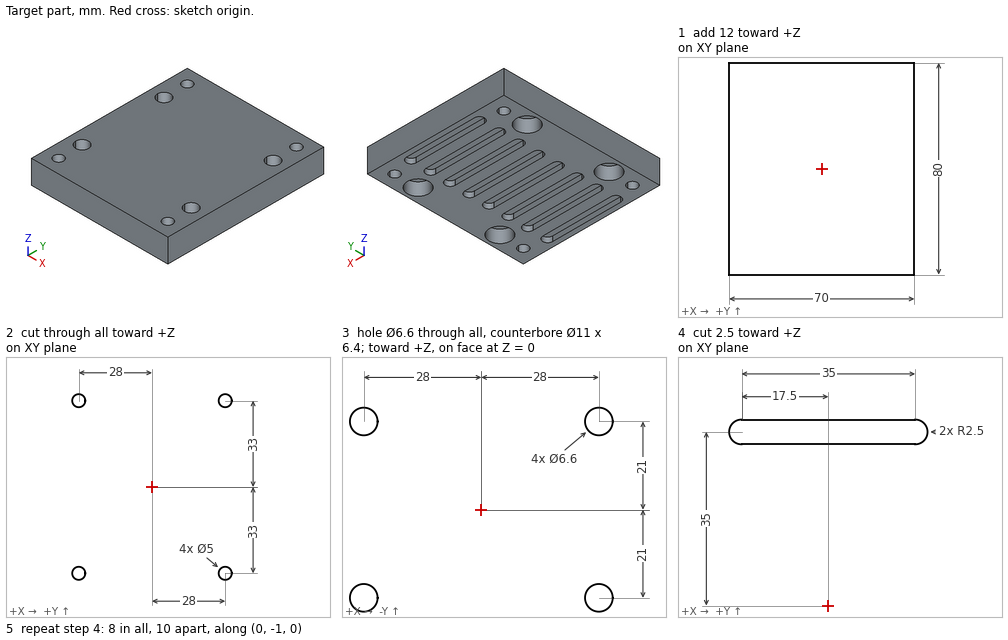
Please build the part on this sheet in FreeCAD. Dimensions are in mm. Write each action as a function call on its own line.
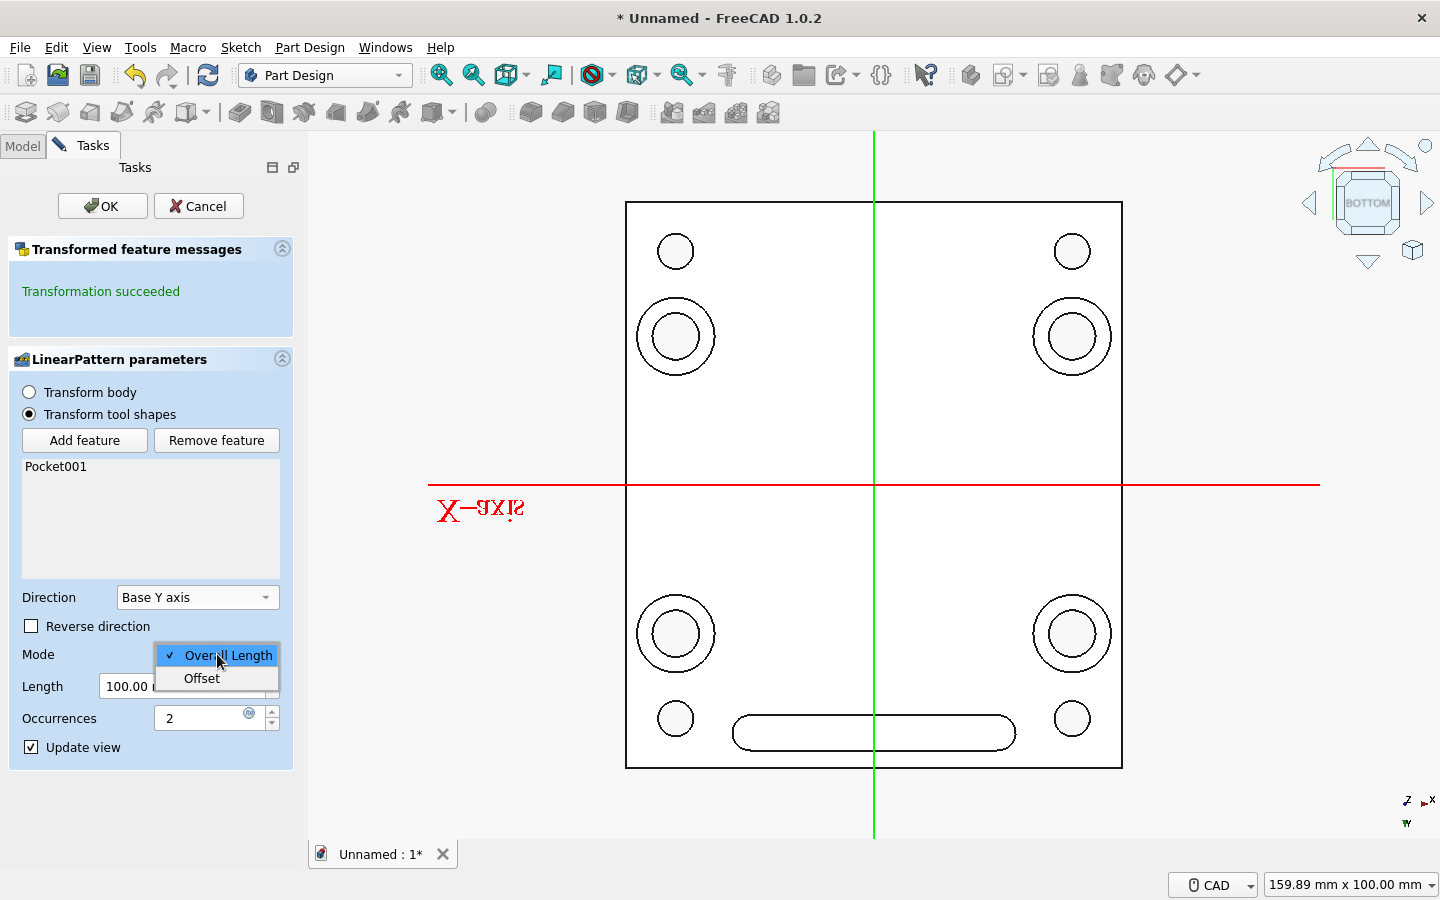
click(216, 678)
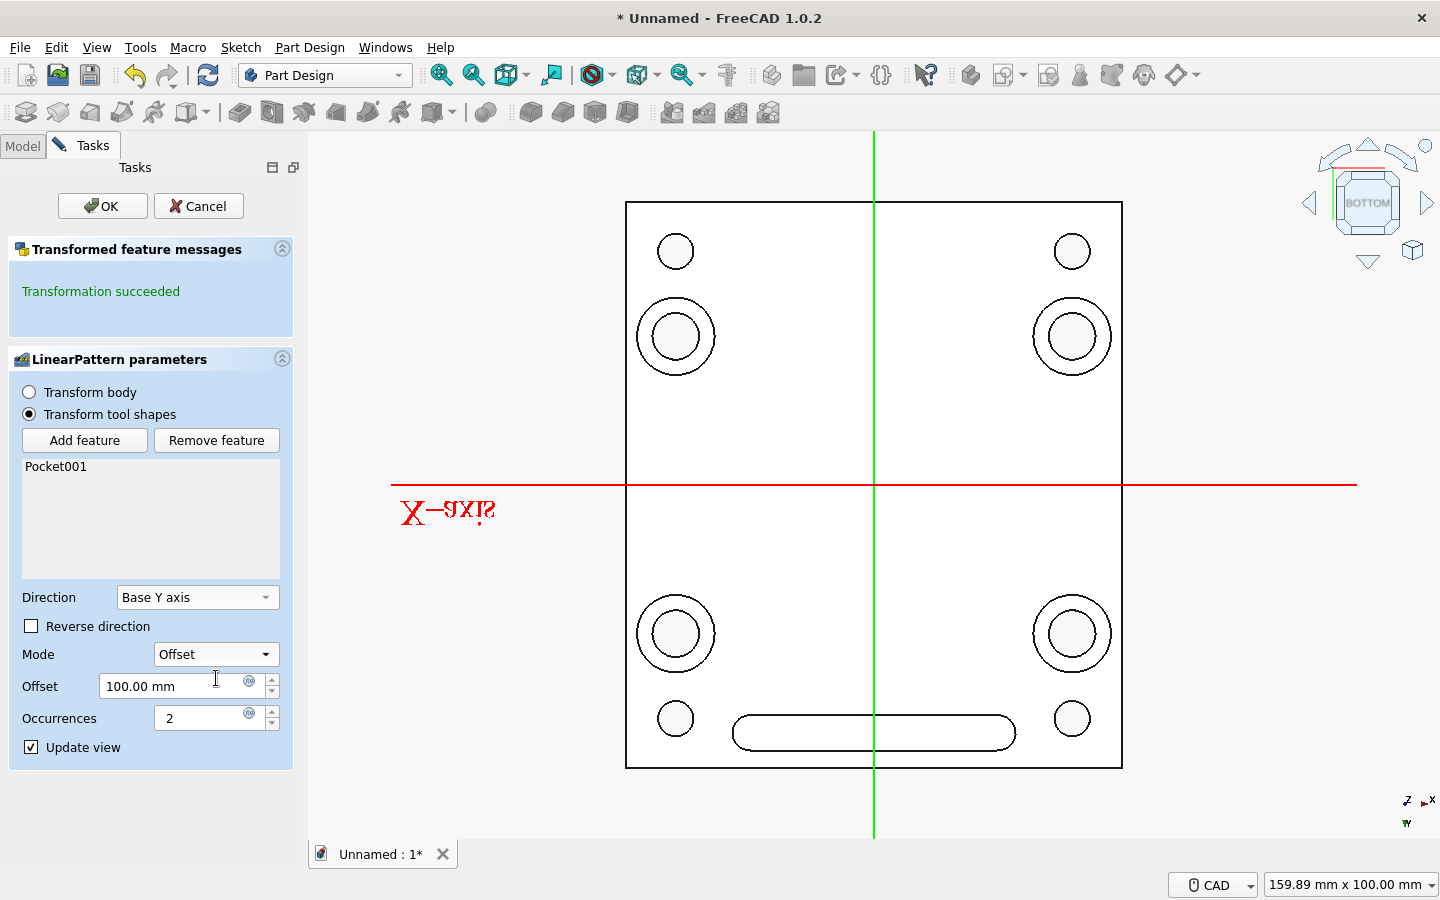
triple_click(182, 686)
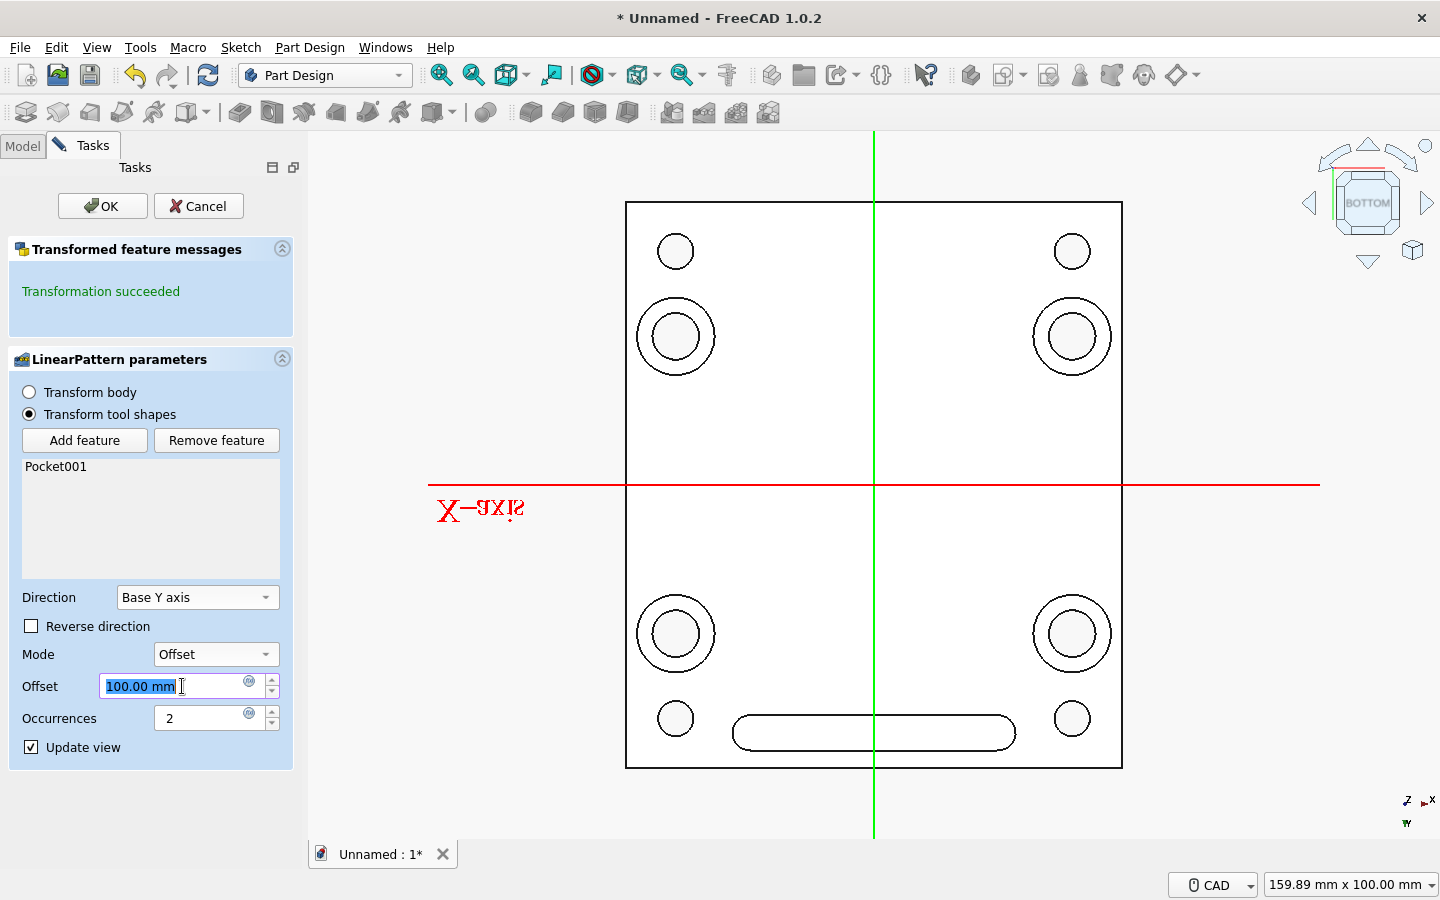
text(10)
key(Tab)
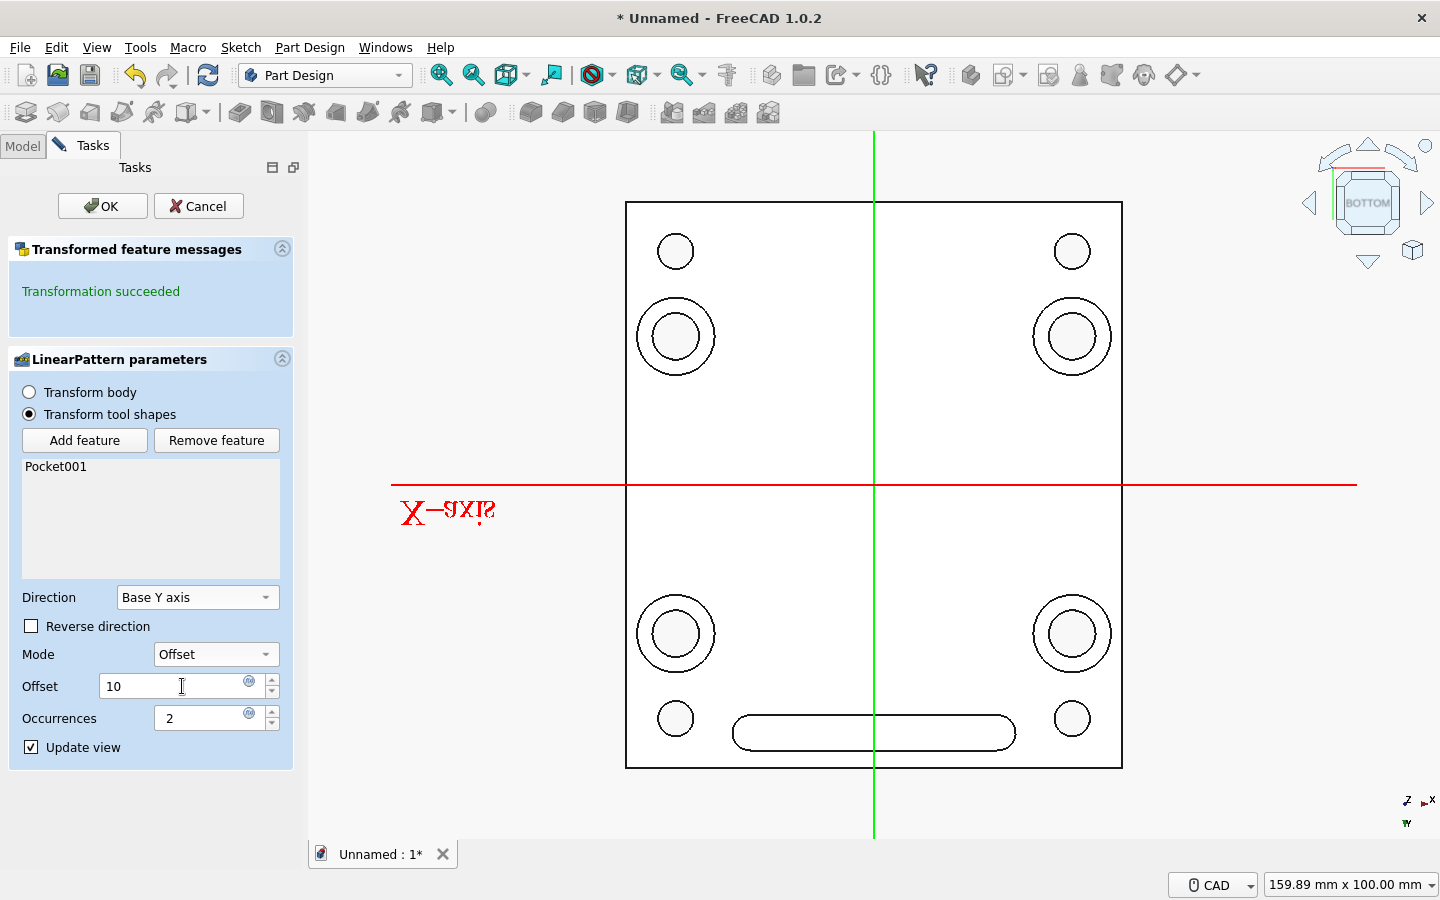
triple_click(209, 718)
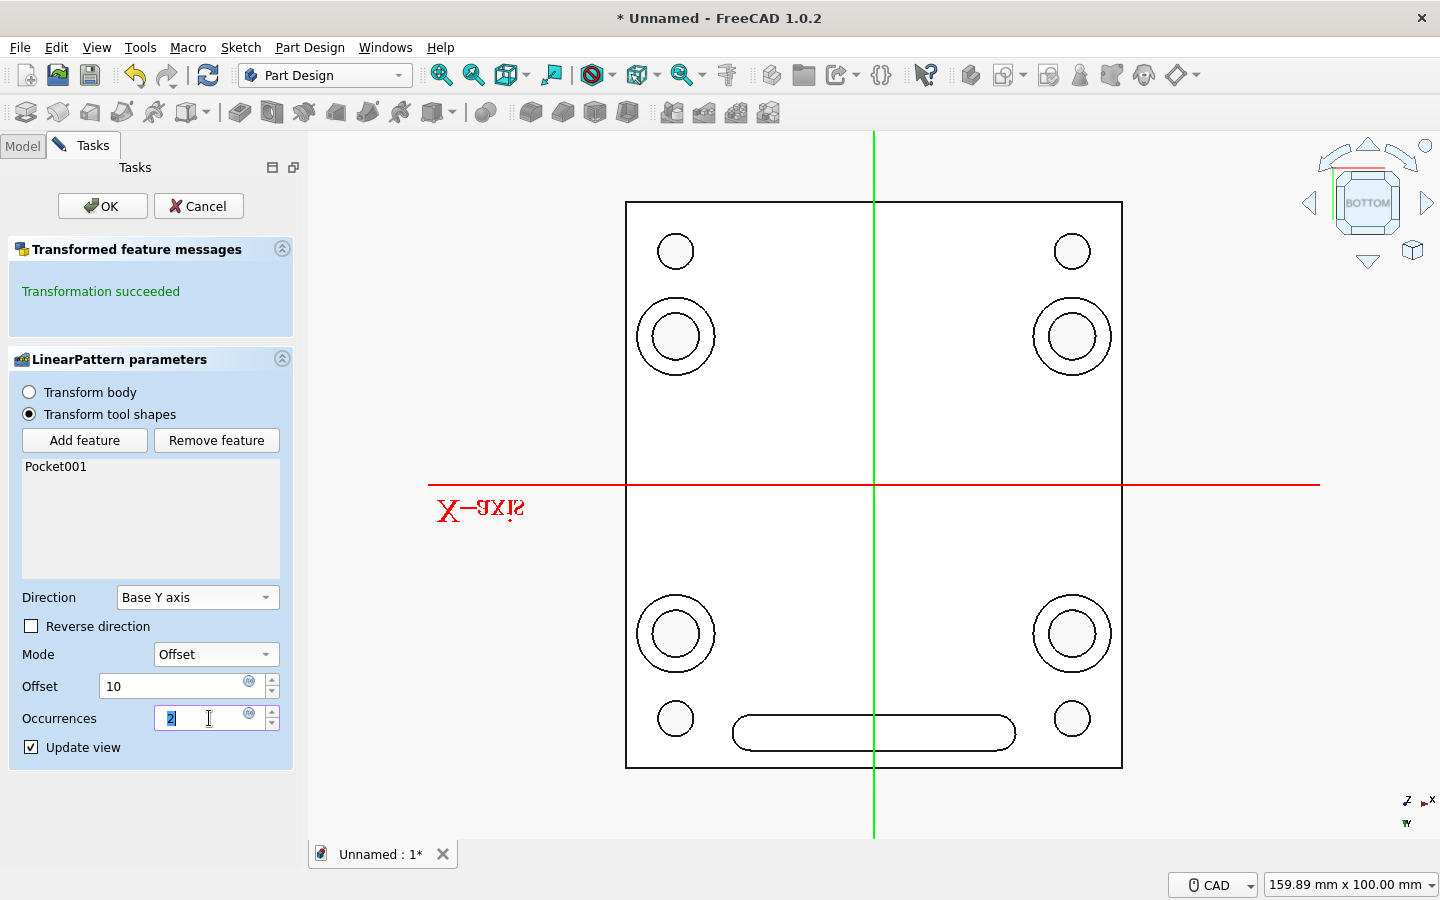
text(8)
key(Tab)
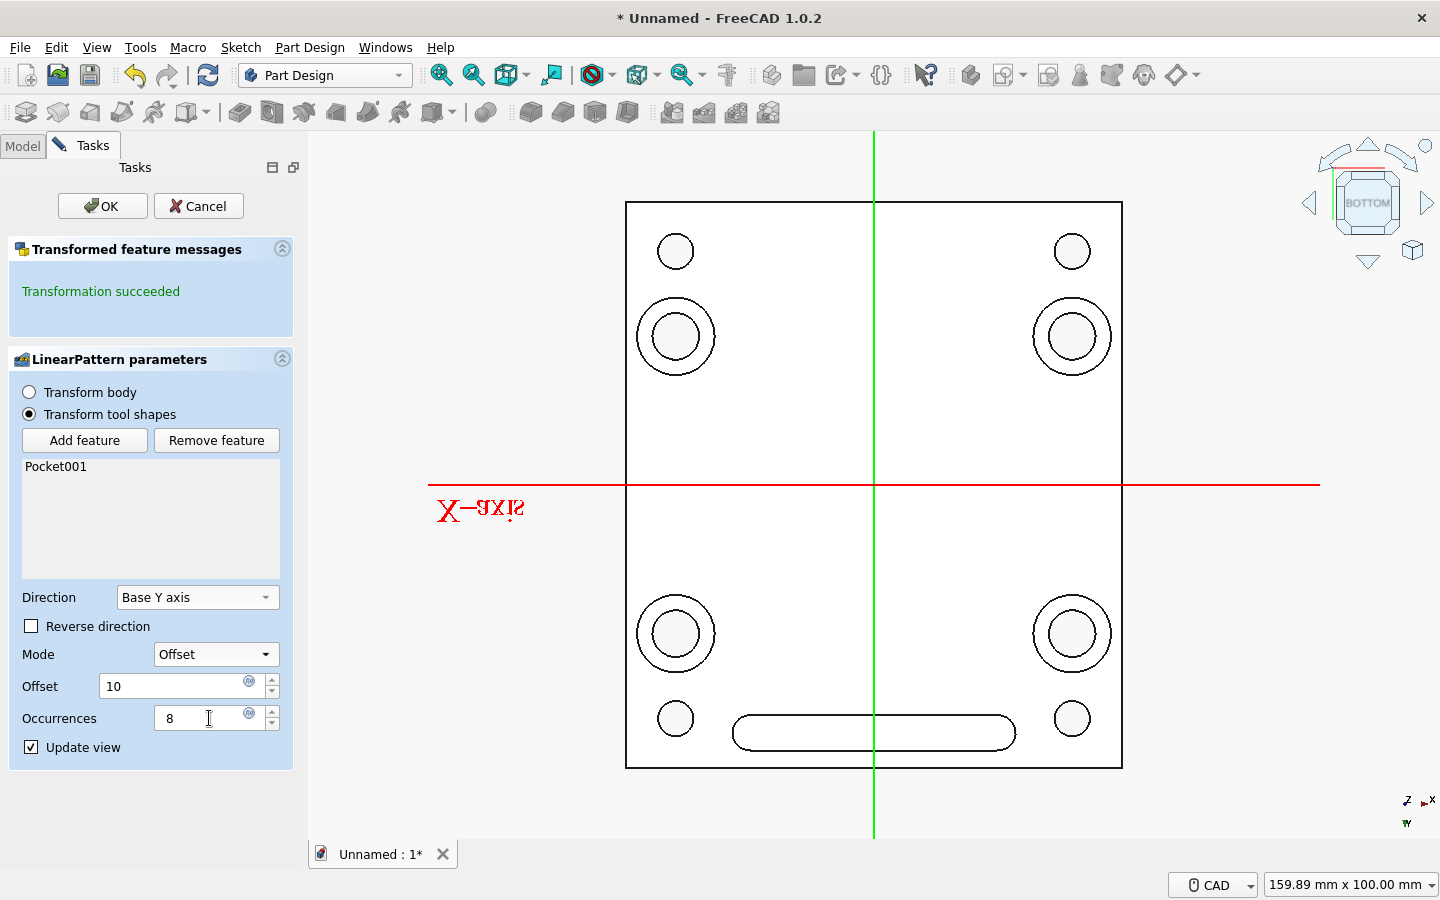
click(30, 626)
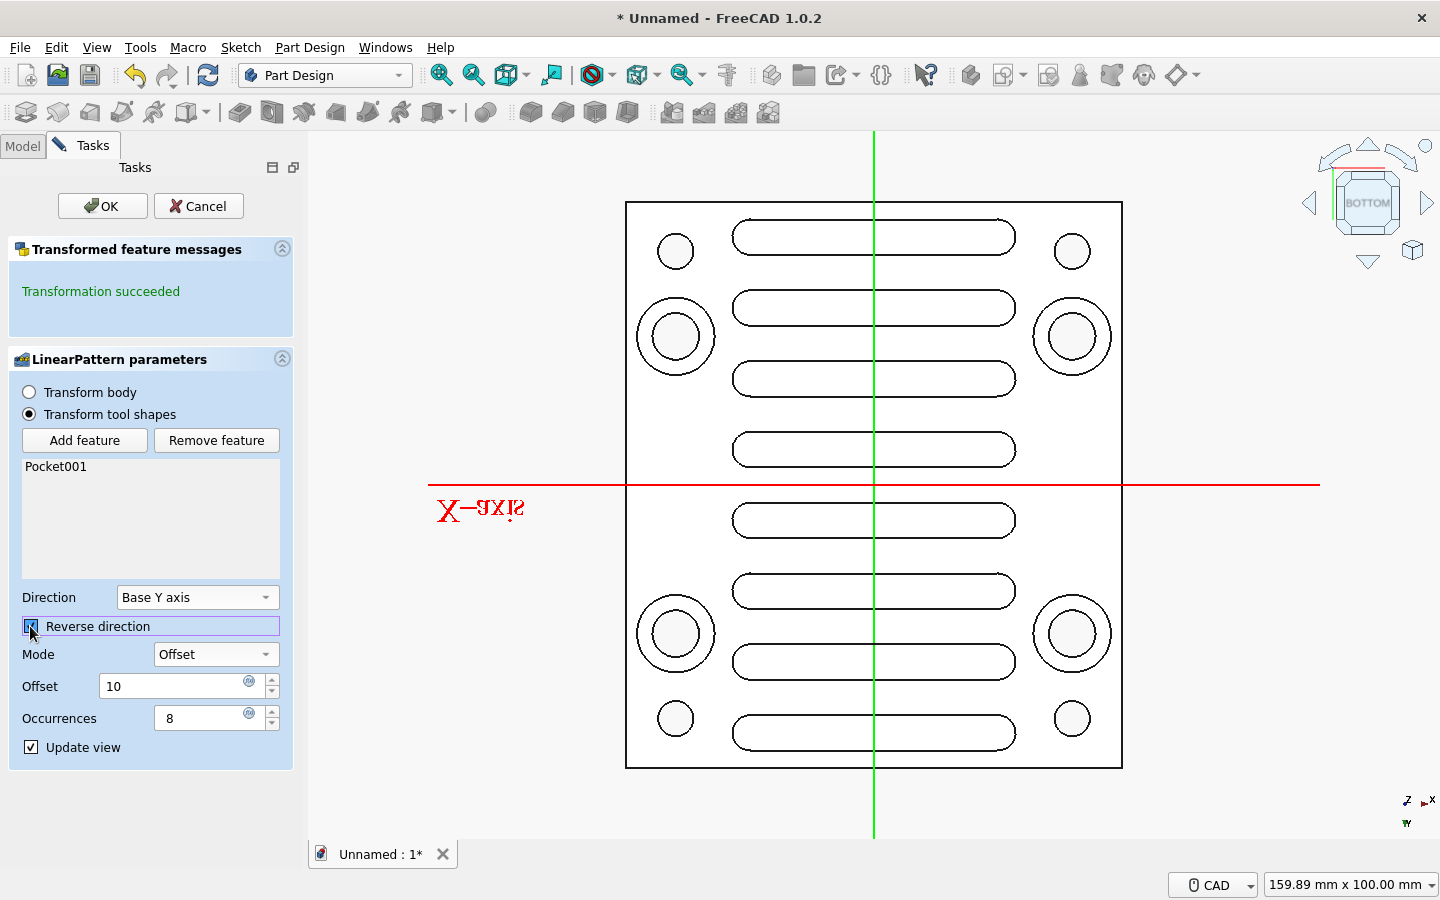
click(103, 206)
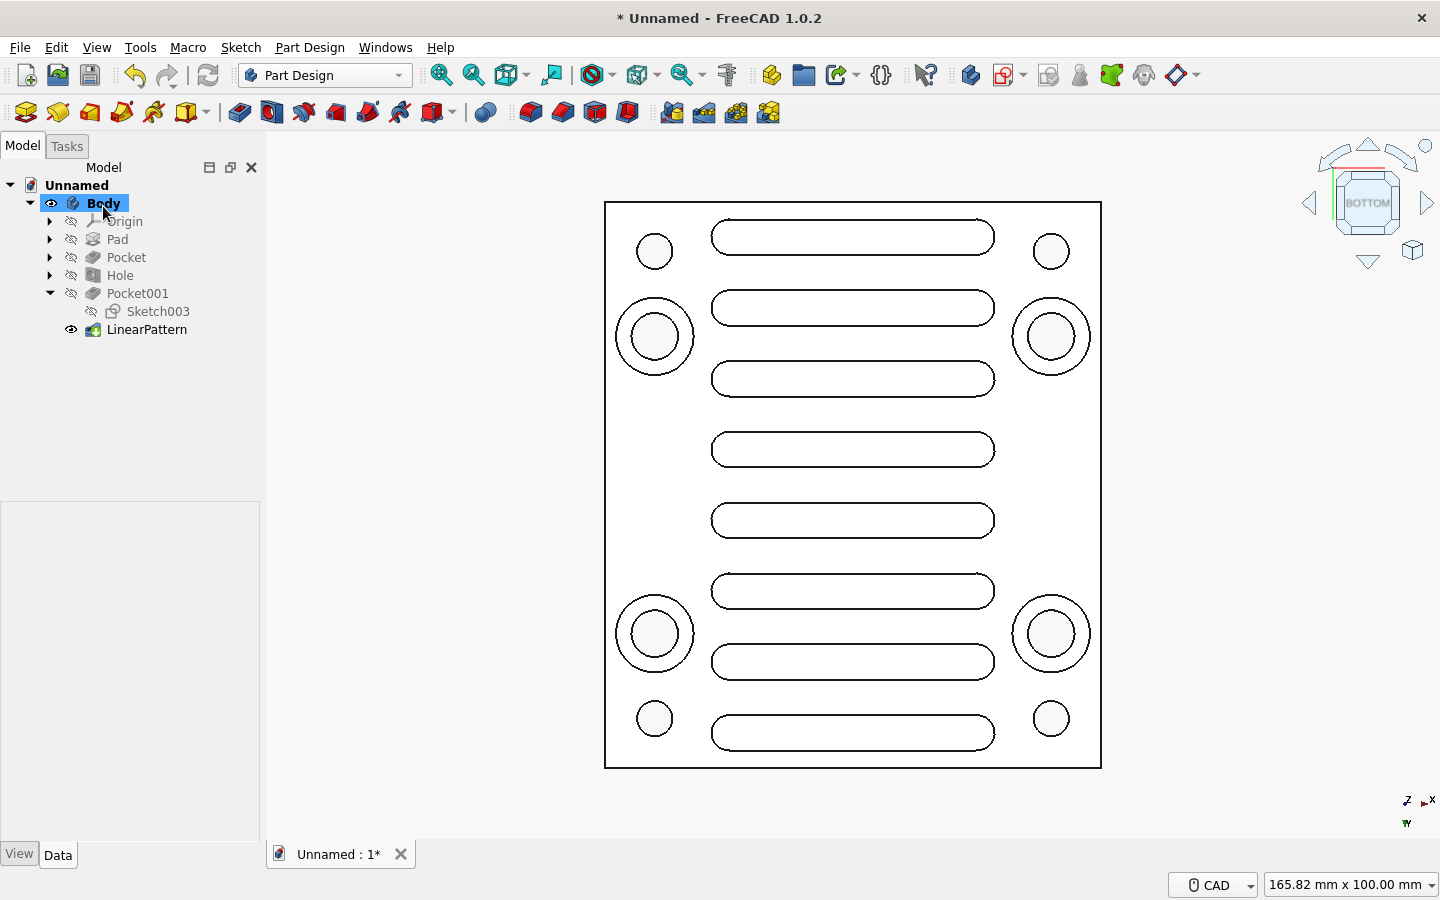
key(0)